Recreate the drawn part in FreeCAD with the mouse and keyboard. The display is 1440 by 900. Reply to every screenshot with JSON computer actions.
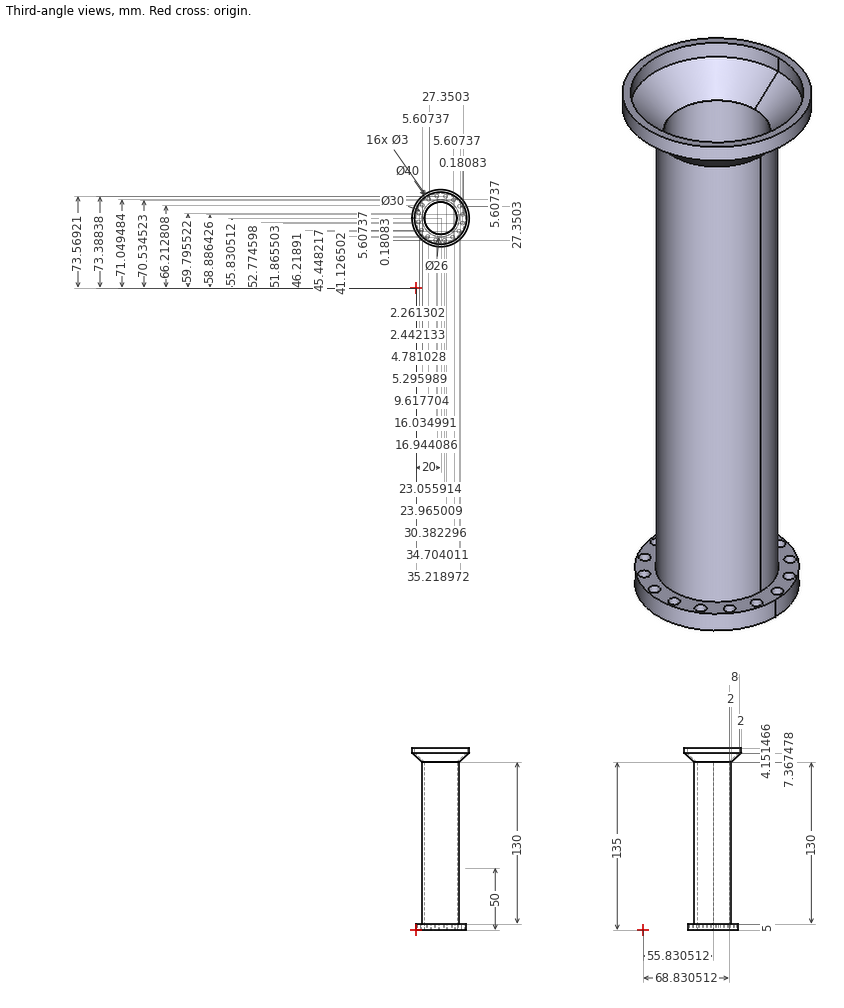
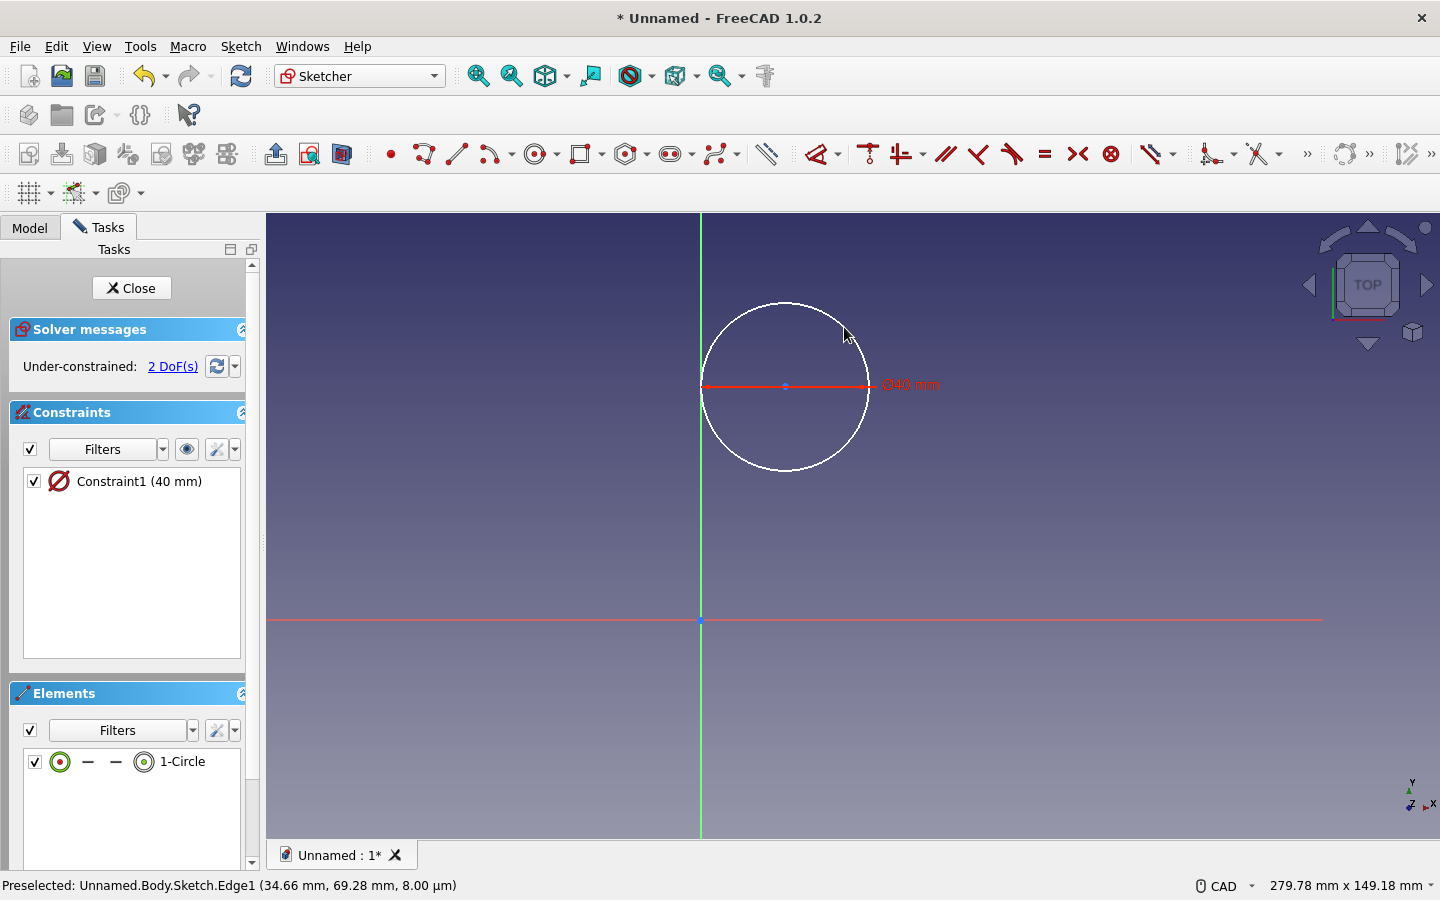
{"action": "left_click", "coordinate": [816, 154]}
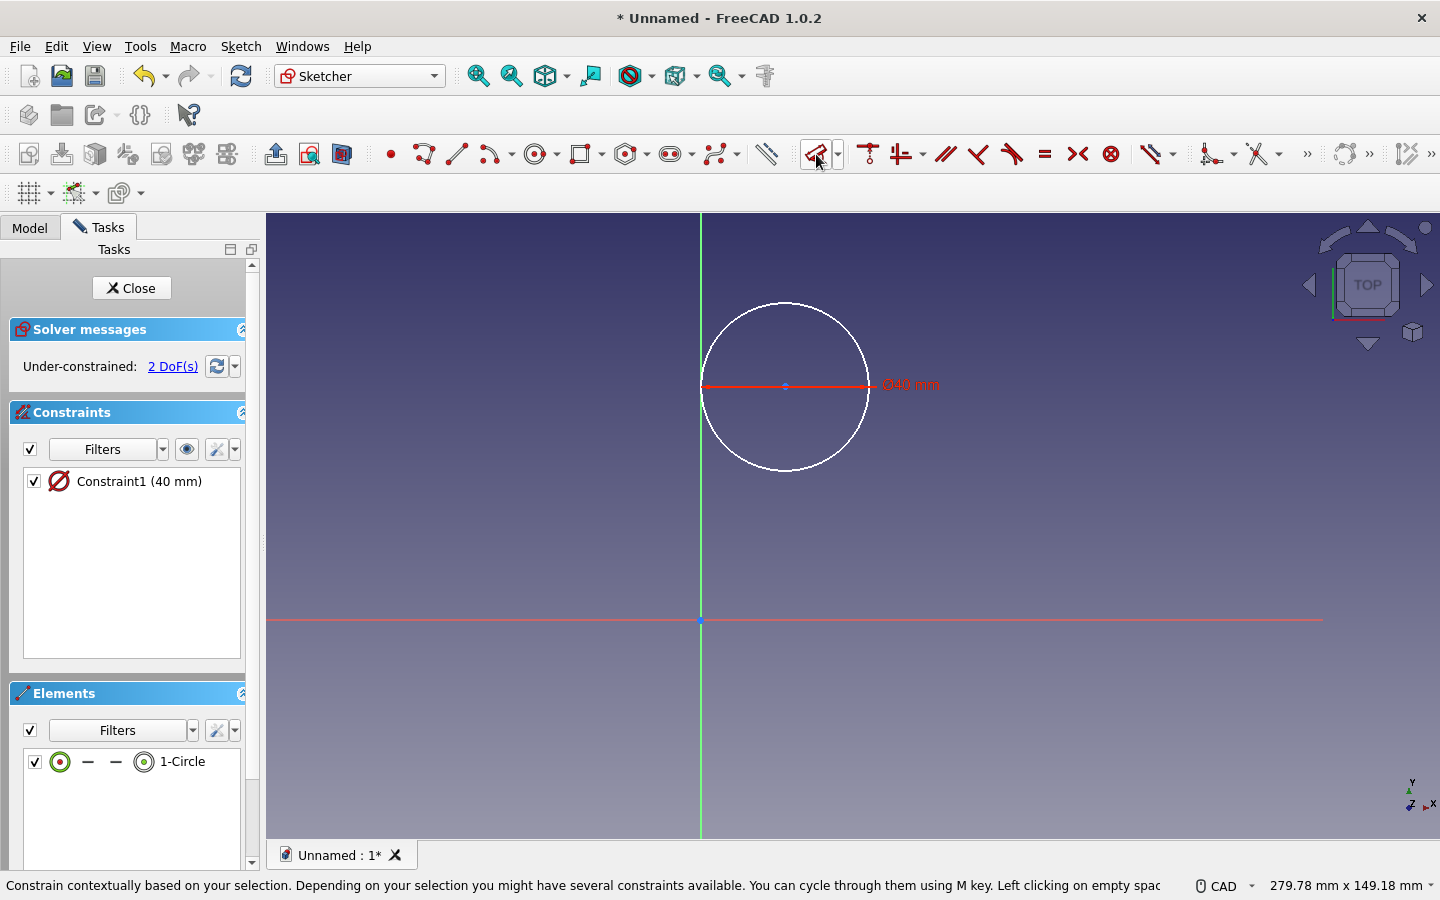
{"action": "left_click", "coordinate": [785, 387]}
{"action": "left_click", "coordinate": [743, 654]}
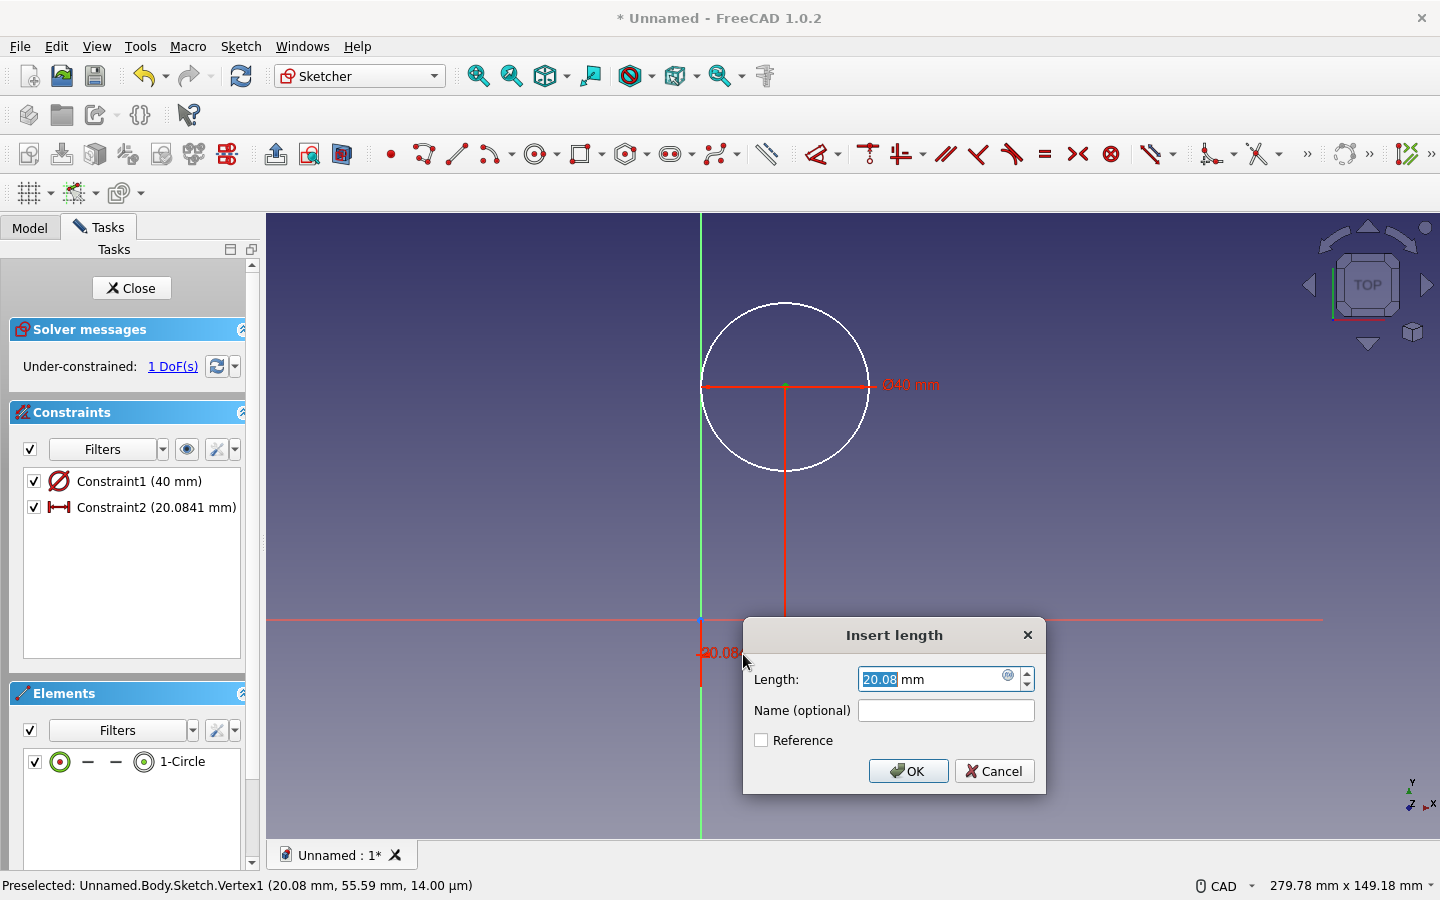
{"action": "type", "text": "20"}
{"action": "key", "text": "Return"}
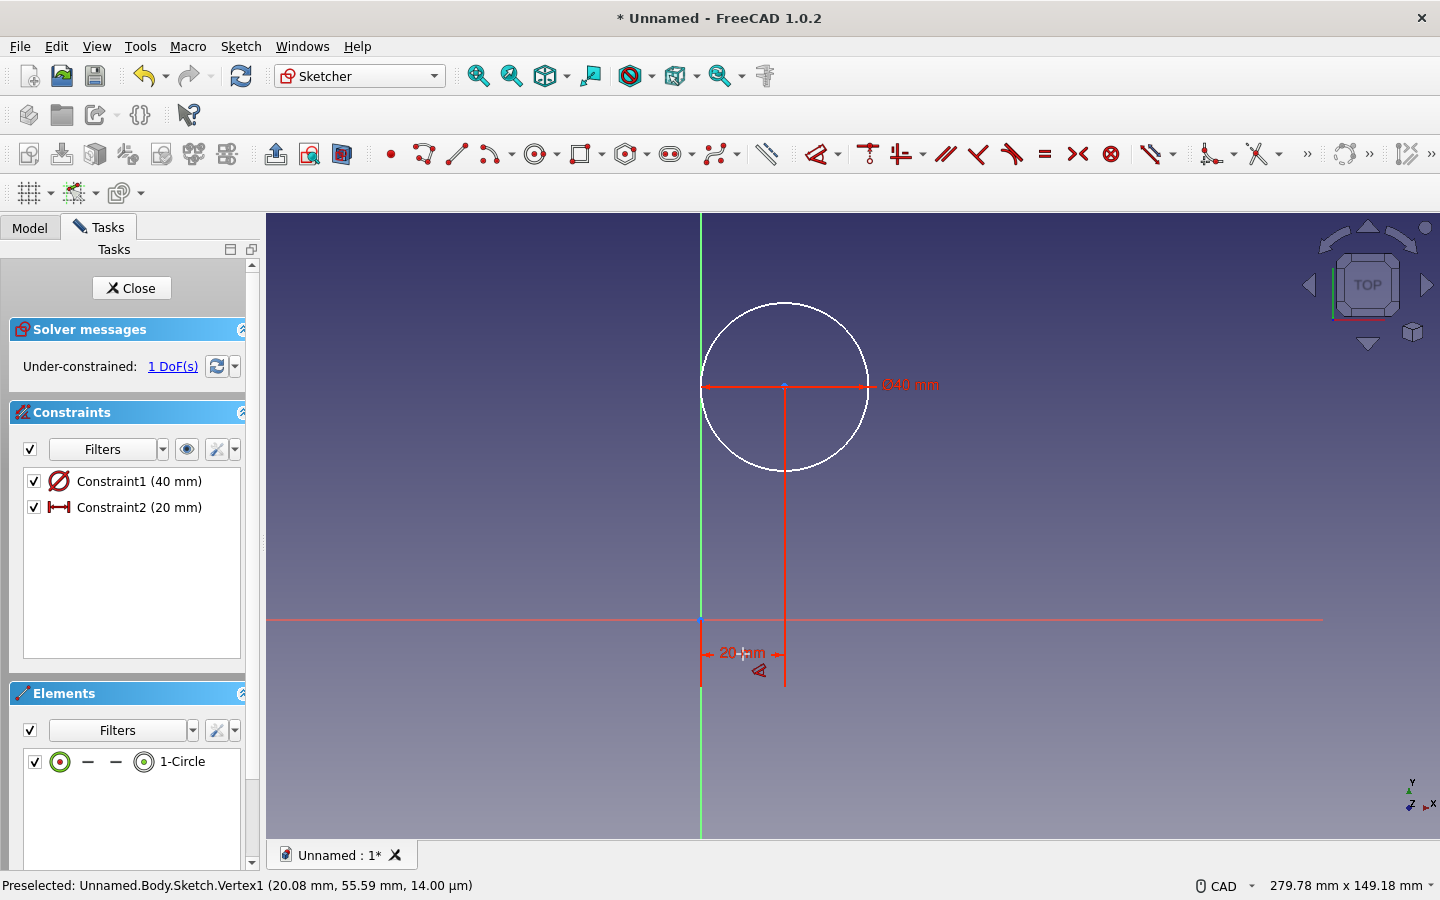
{"action": "left_click", "coordinate": [785, 387]}
{"action": "left_click", "coordinate": [667, 504]}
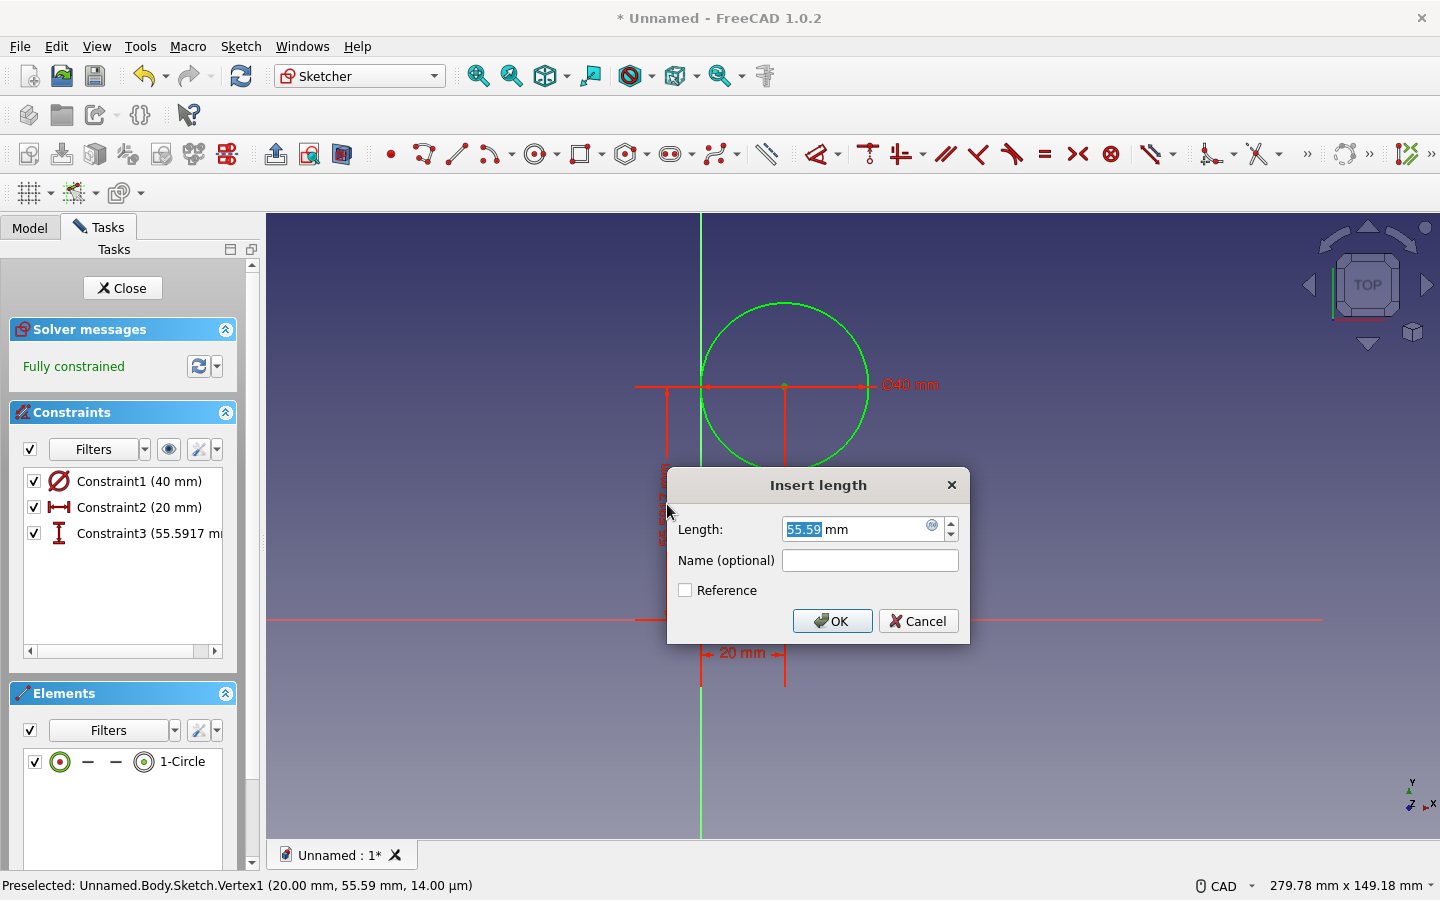
{"action": "type", "text": "55.830512"}
{"action": "key", "text": "Return"}
{"action": "key", "text": "Escape"}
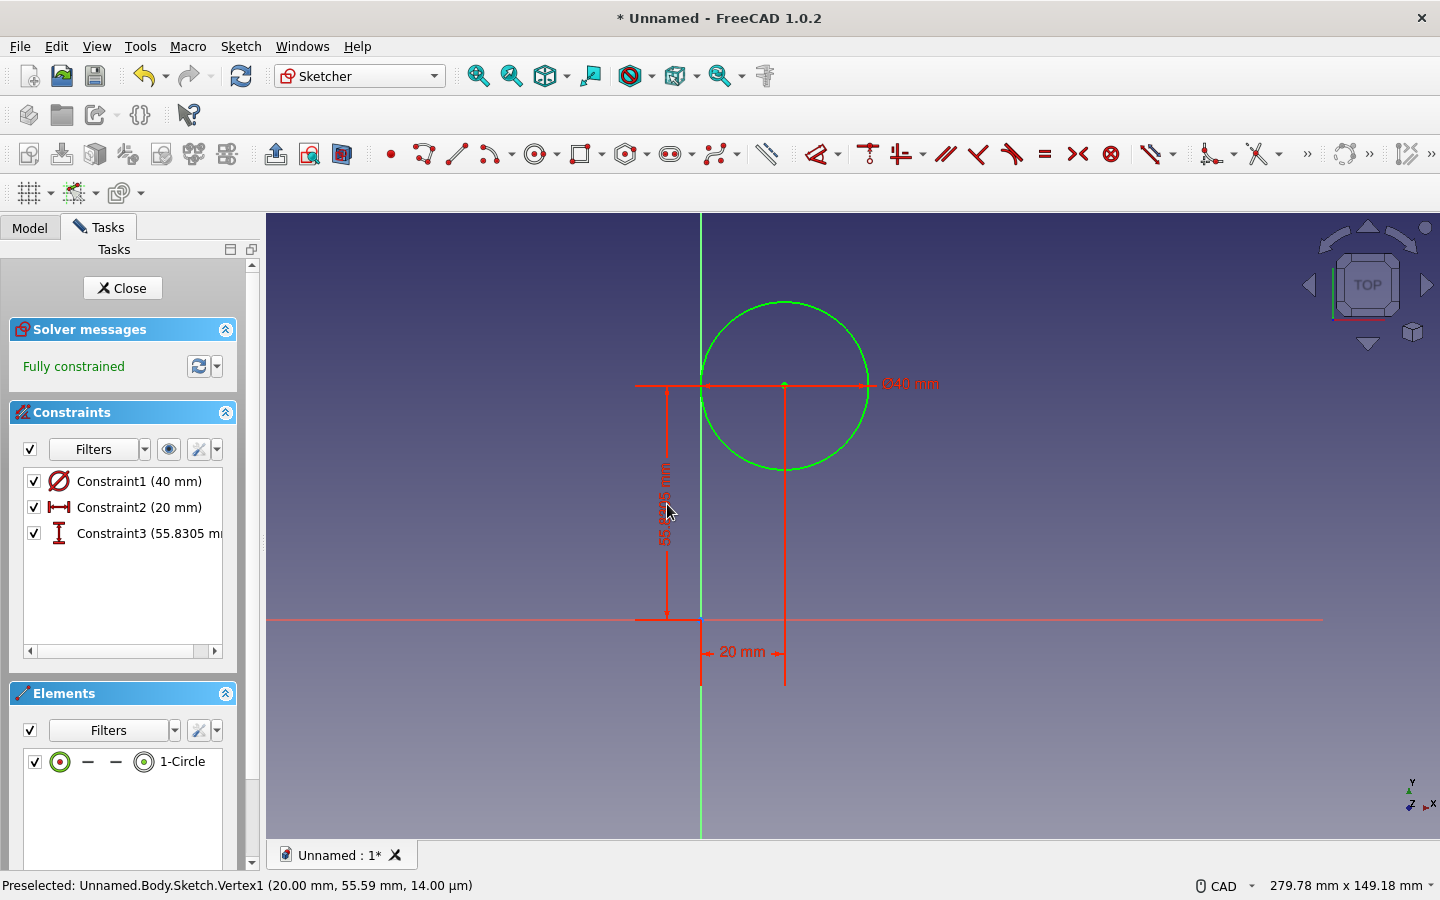
{"action": "left_click", "coordinate": [123, 288]}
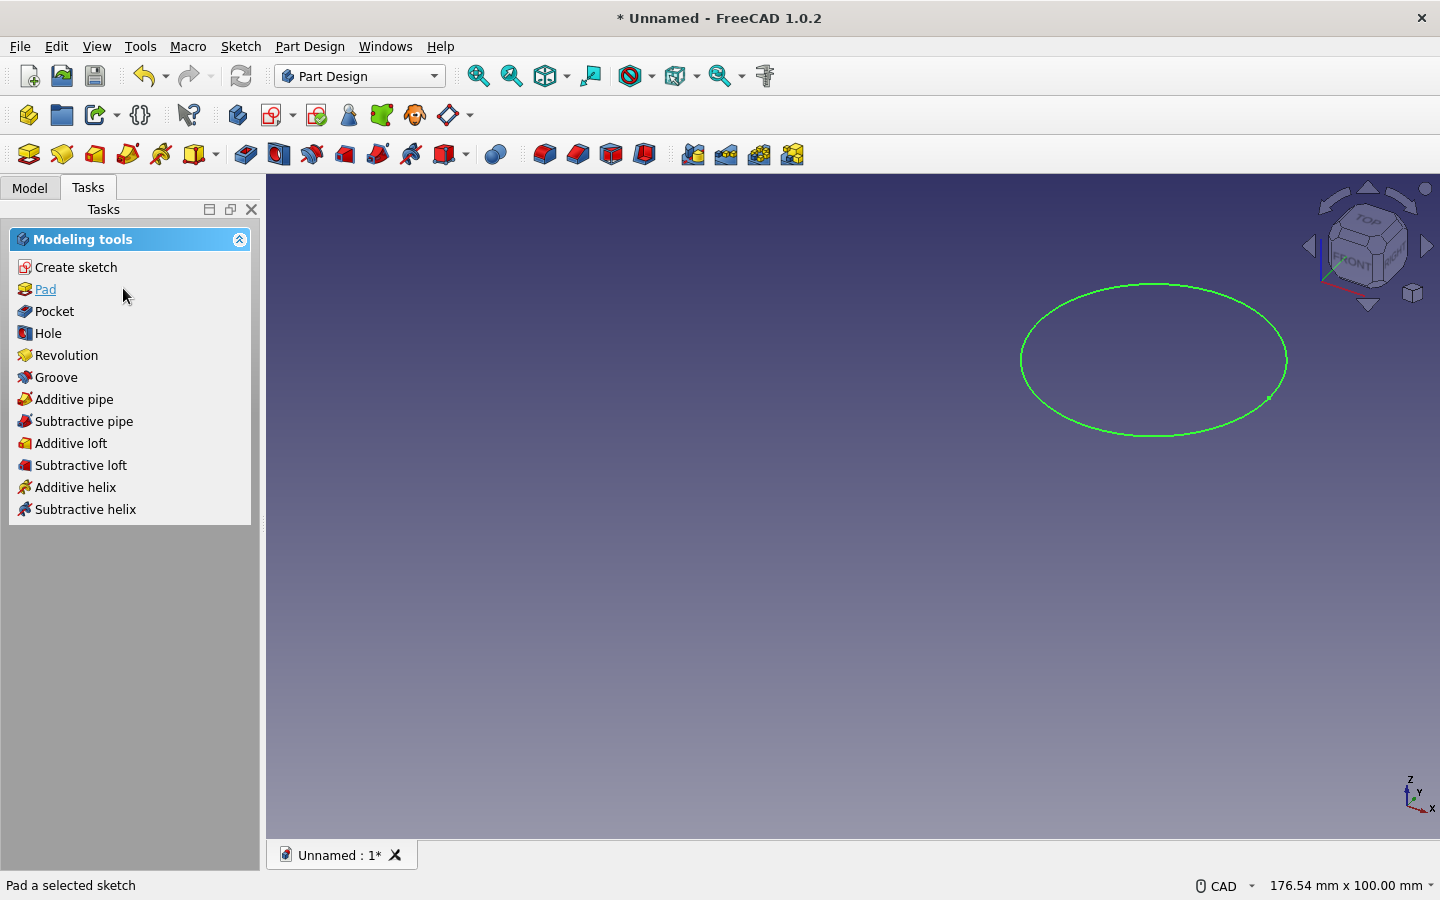
{"action": "left_click", "coordinate": [29, 154]}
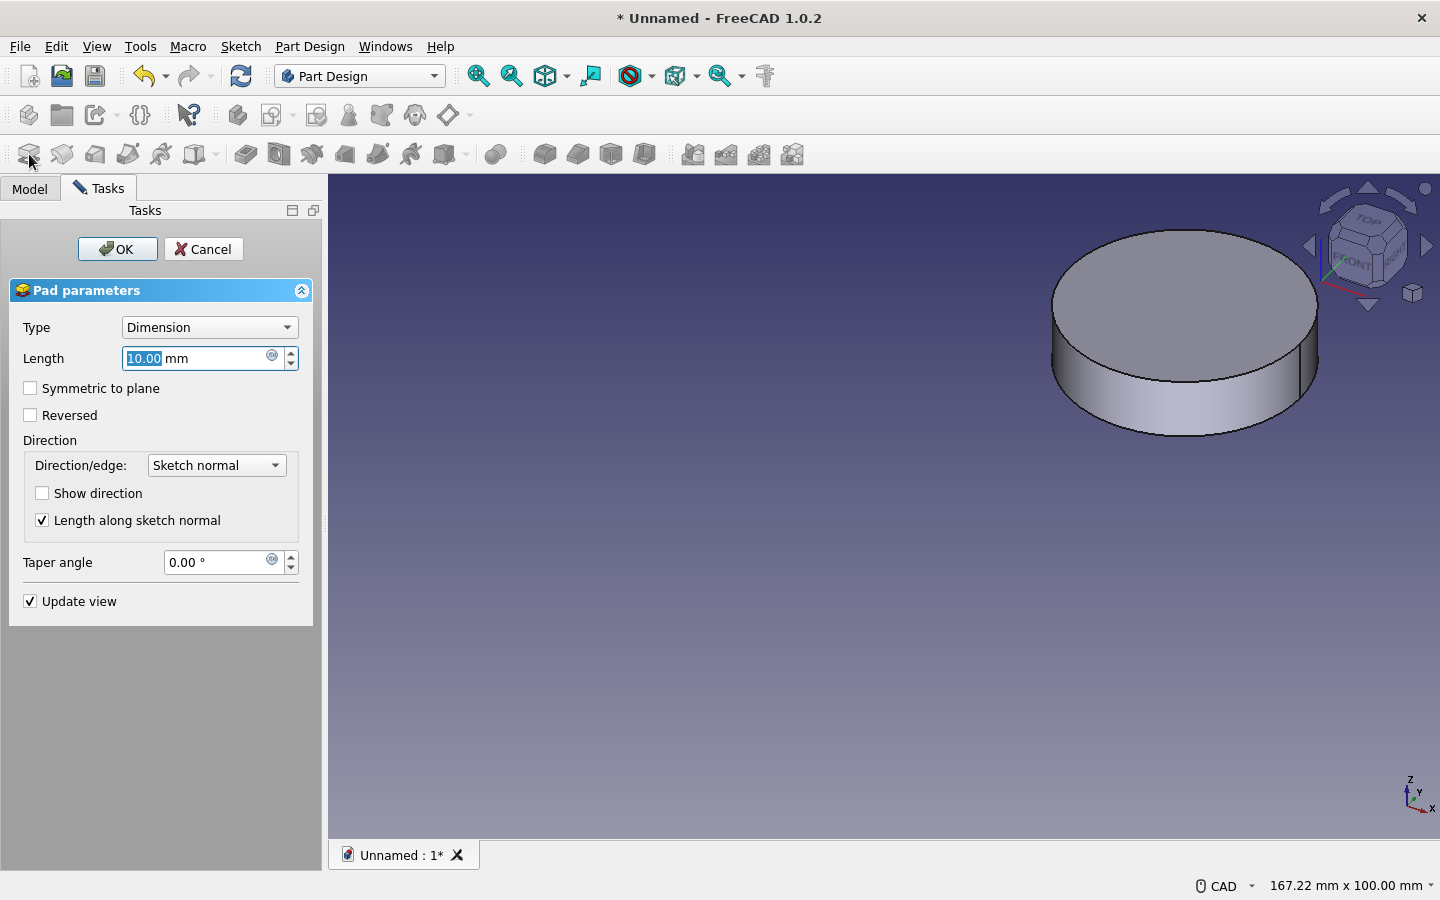
{"action": "type", "text": "5"}
{"action": "key", "text": "Tab"}